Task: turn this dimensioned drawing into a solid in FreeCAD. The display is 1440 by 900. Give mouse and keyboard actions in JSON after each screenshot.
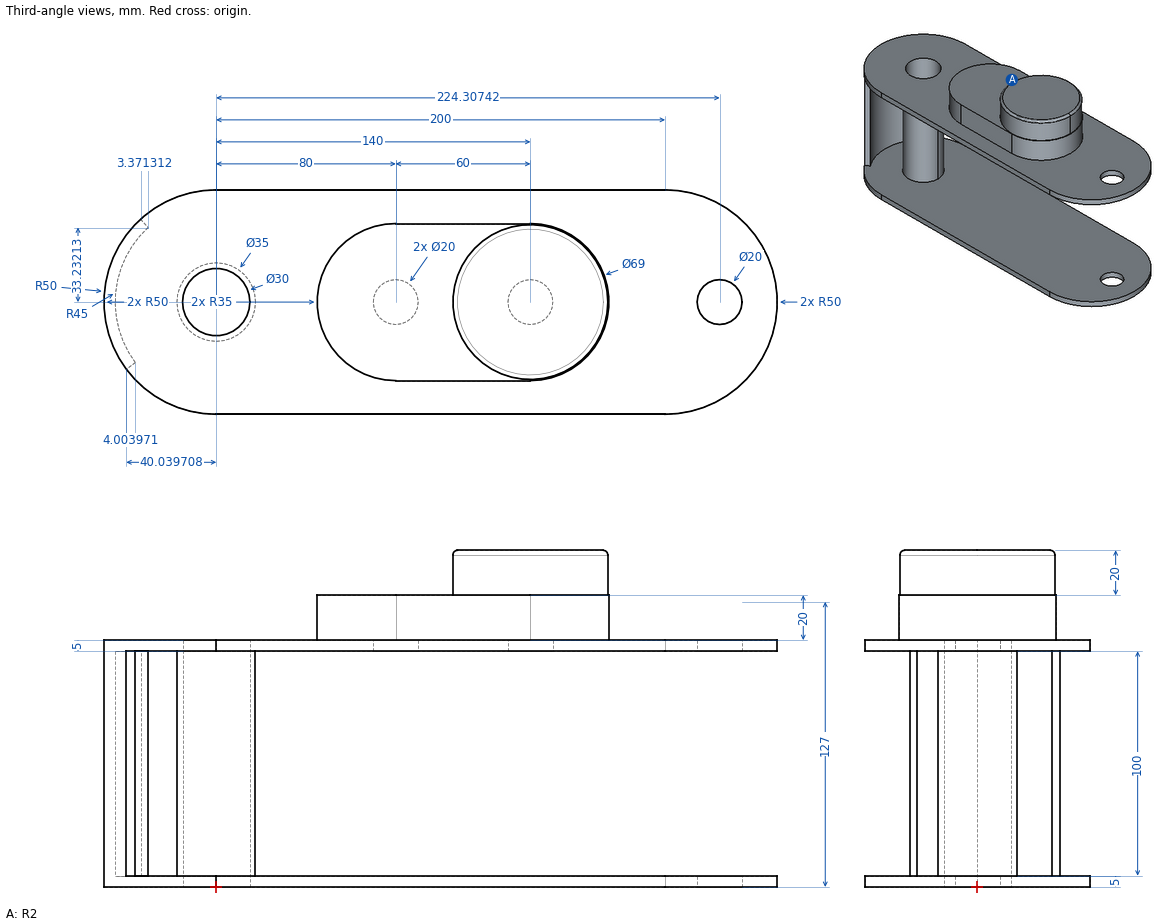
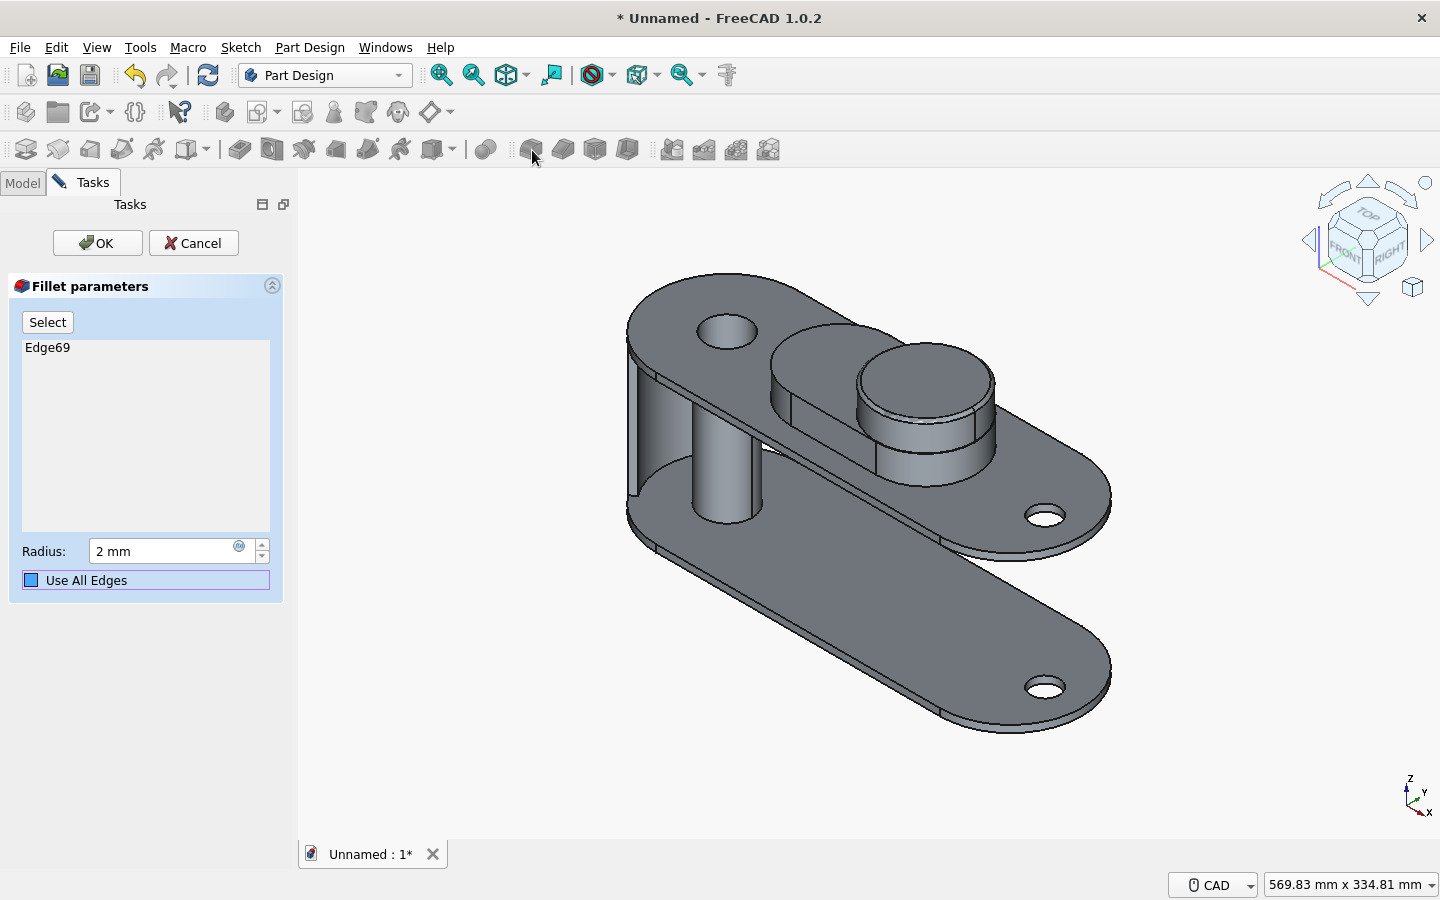
{"action": "left_click", "coordinate": [98, 243]}